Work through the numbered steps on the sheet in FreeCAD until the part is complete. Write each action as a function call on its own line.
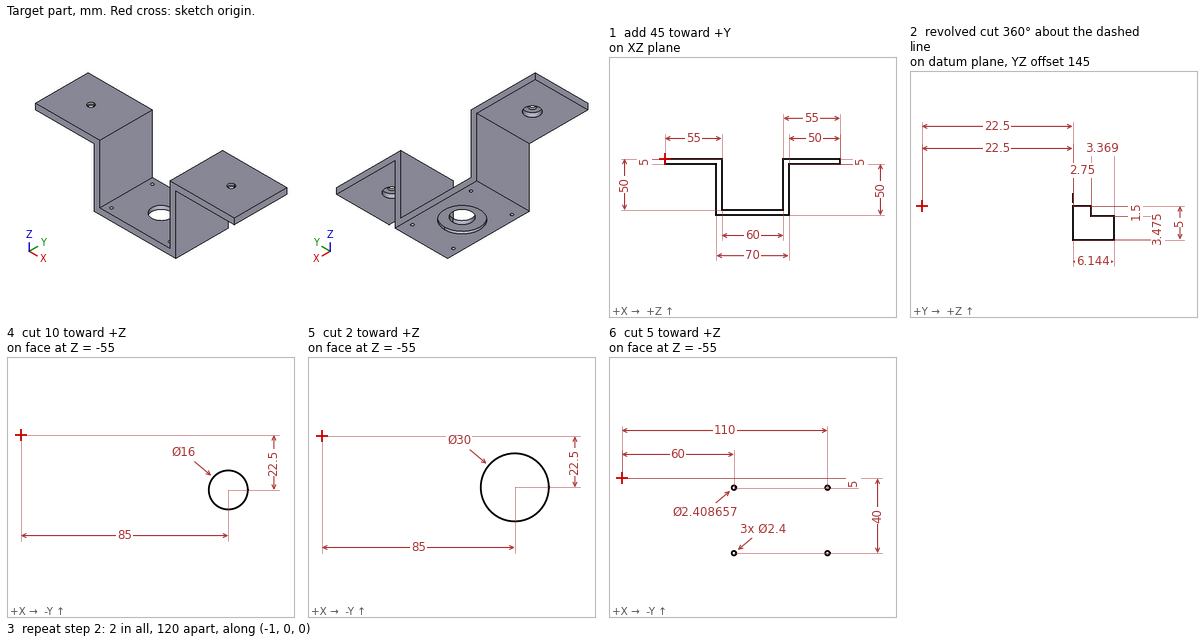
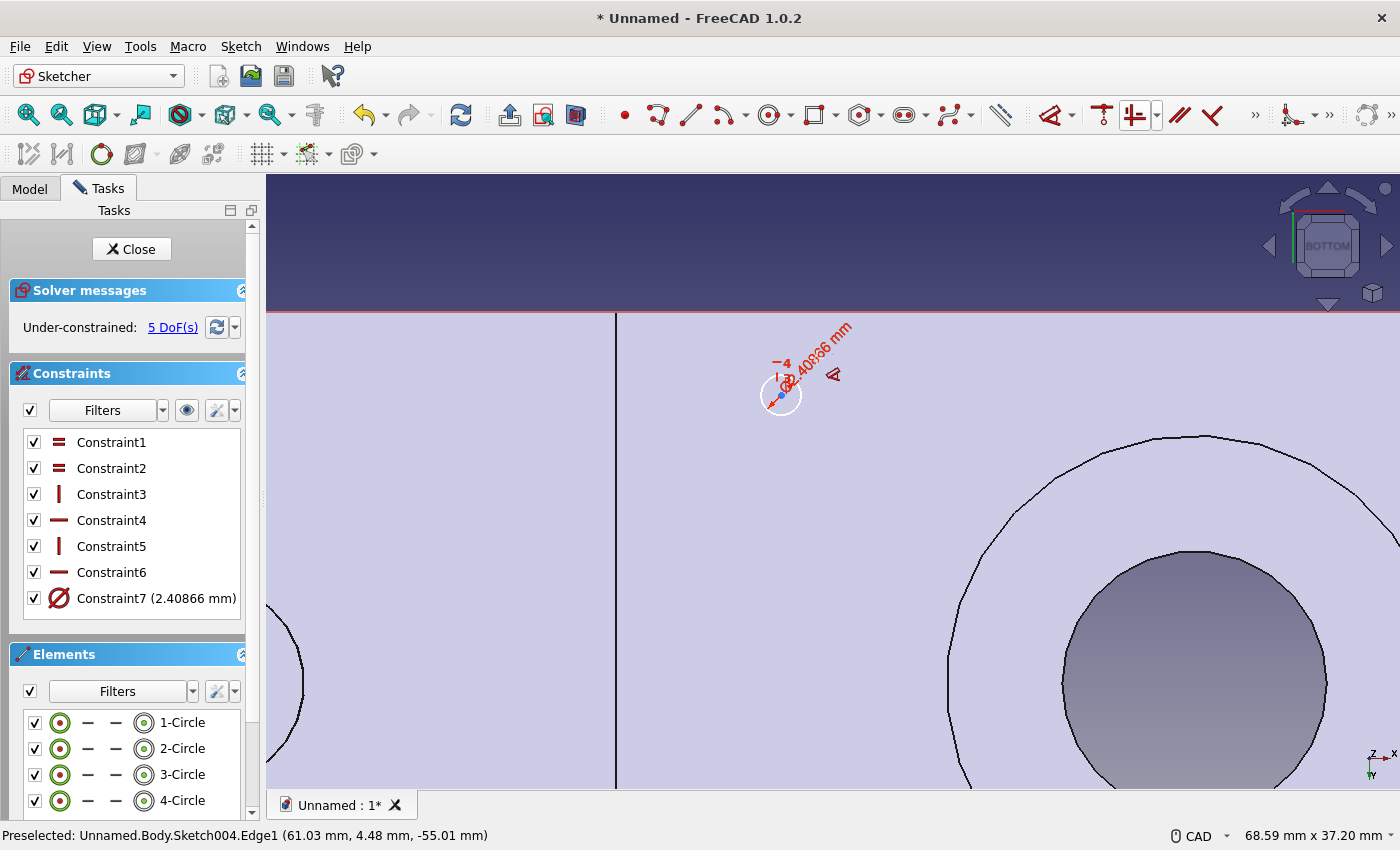
scroll(797, 382, down, 5)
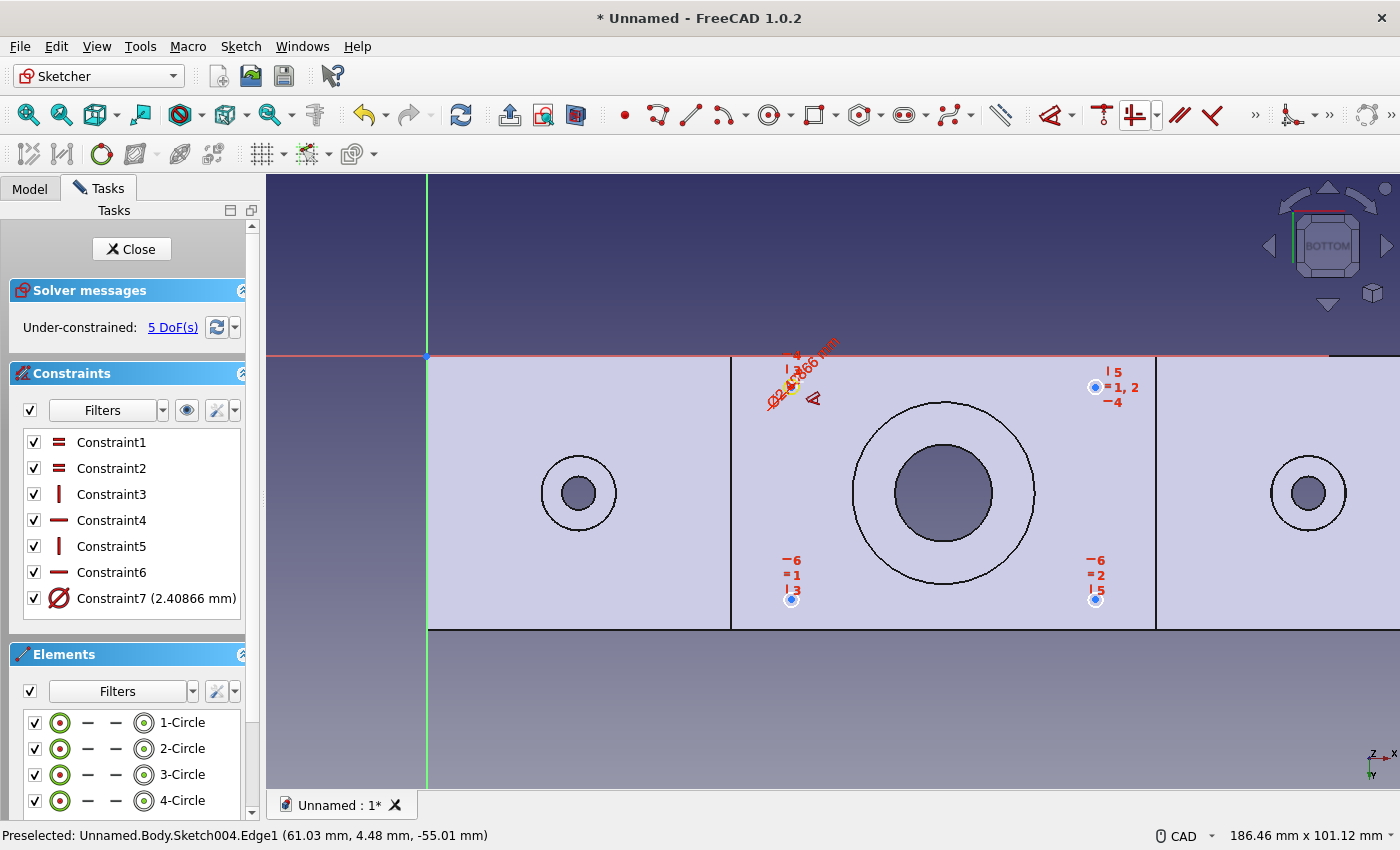
scroll(797, 595, up, 6)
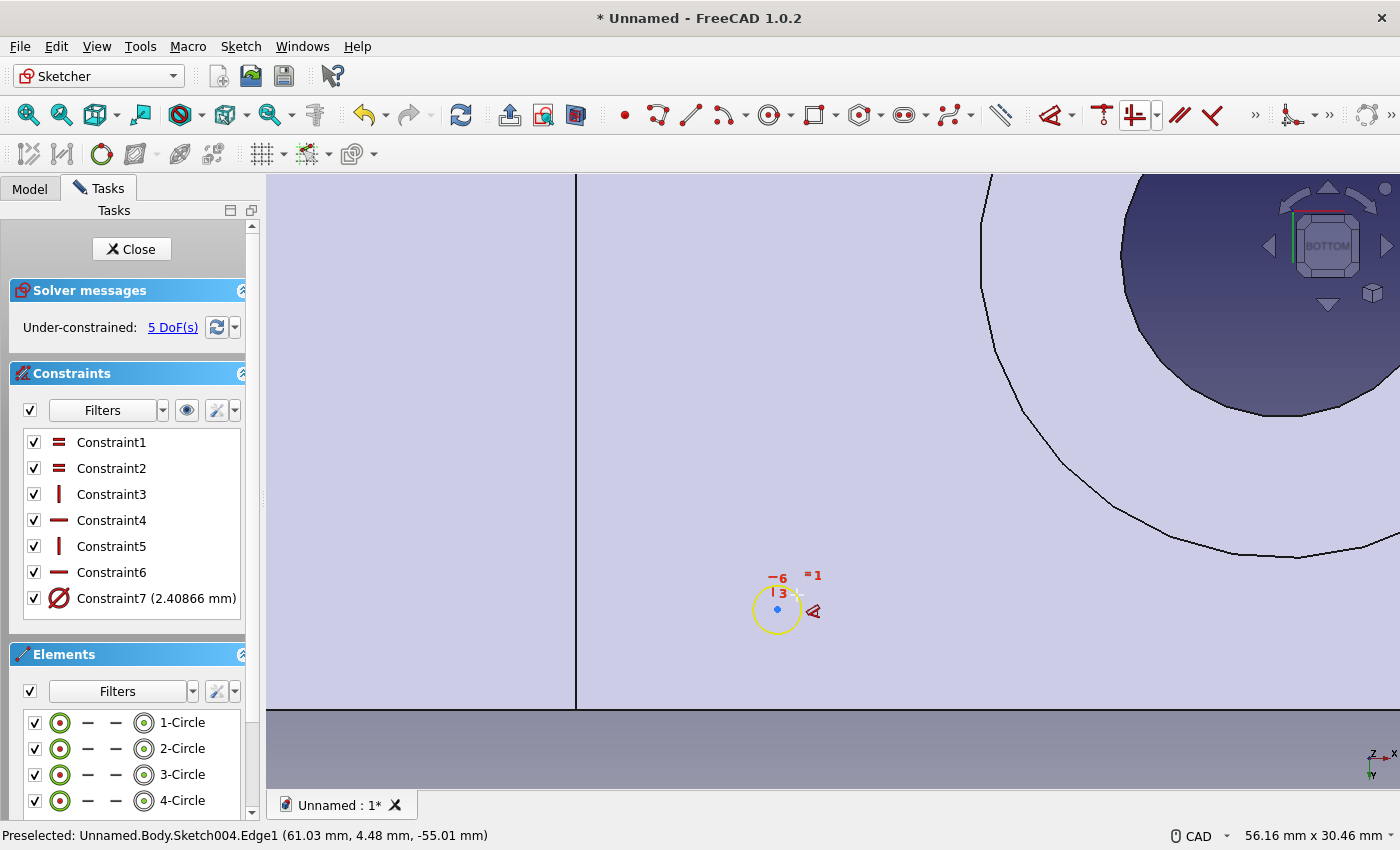
click(794, 593)
click(817, 570)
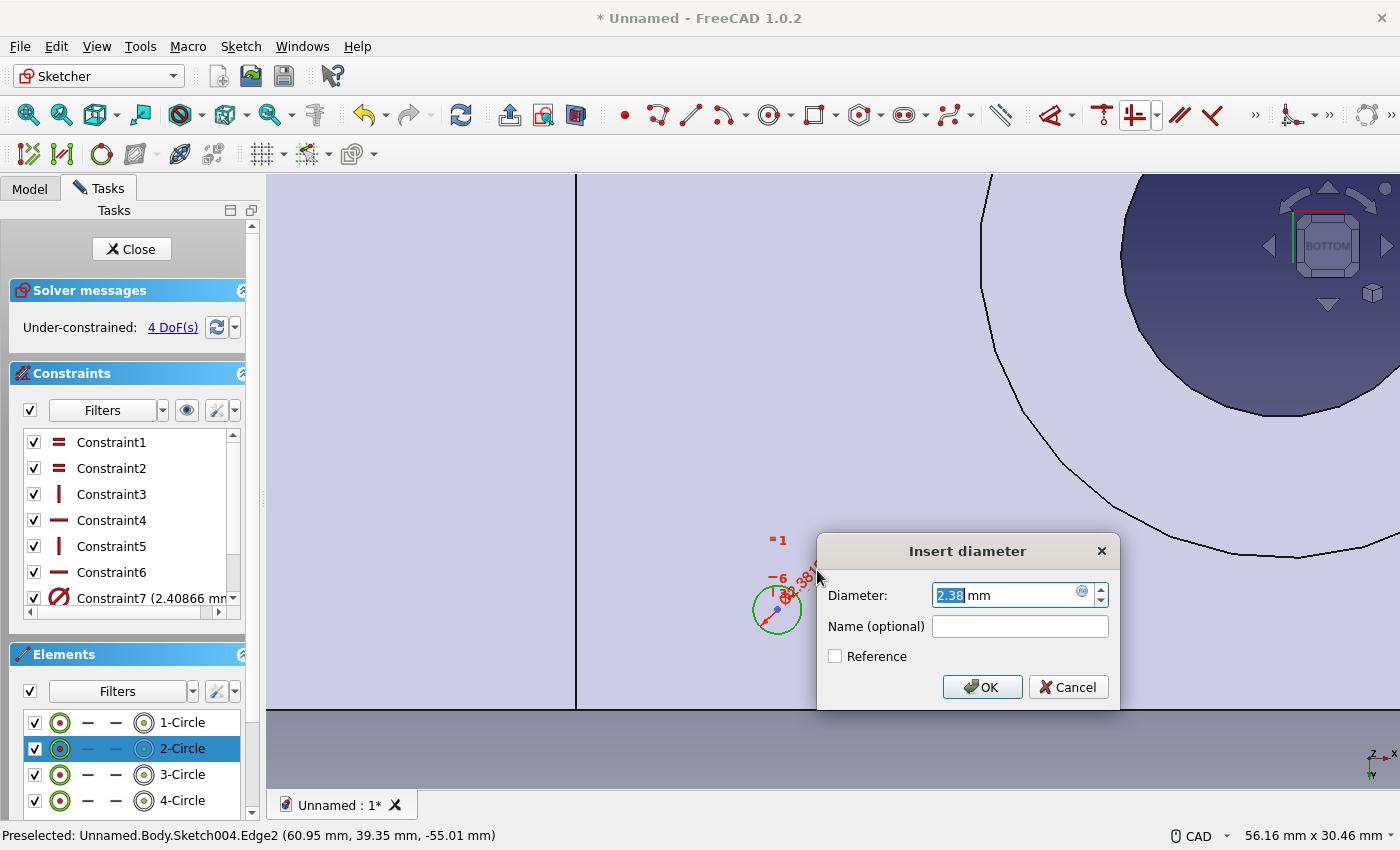
text(2.4)
key(Return)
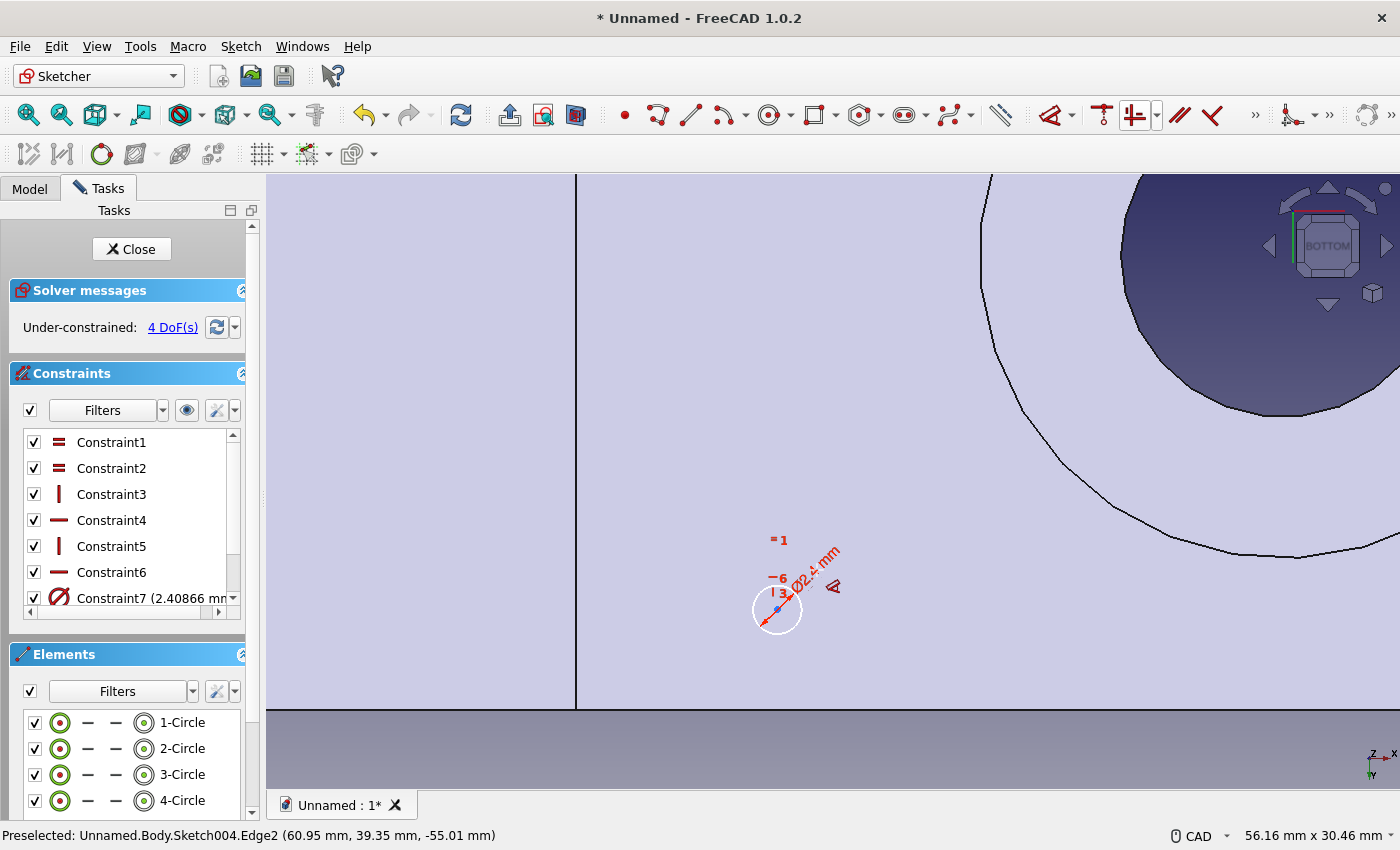
scroll(797, 596, down, 6)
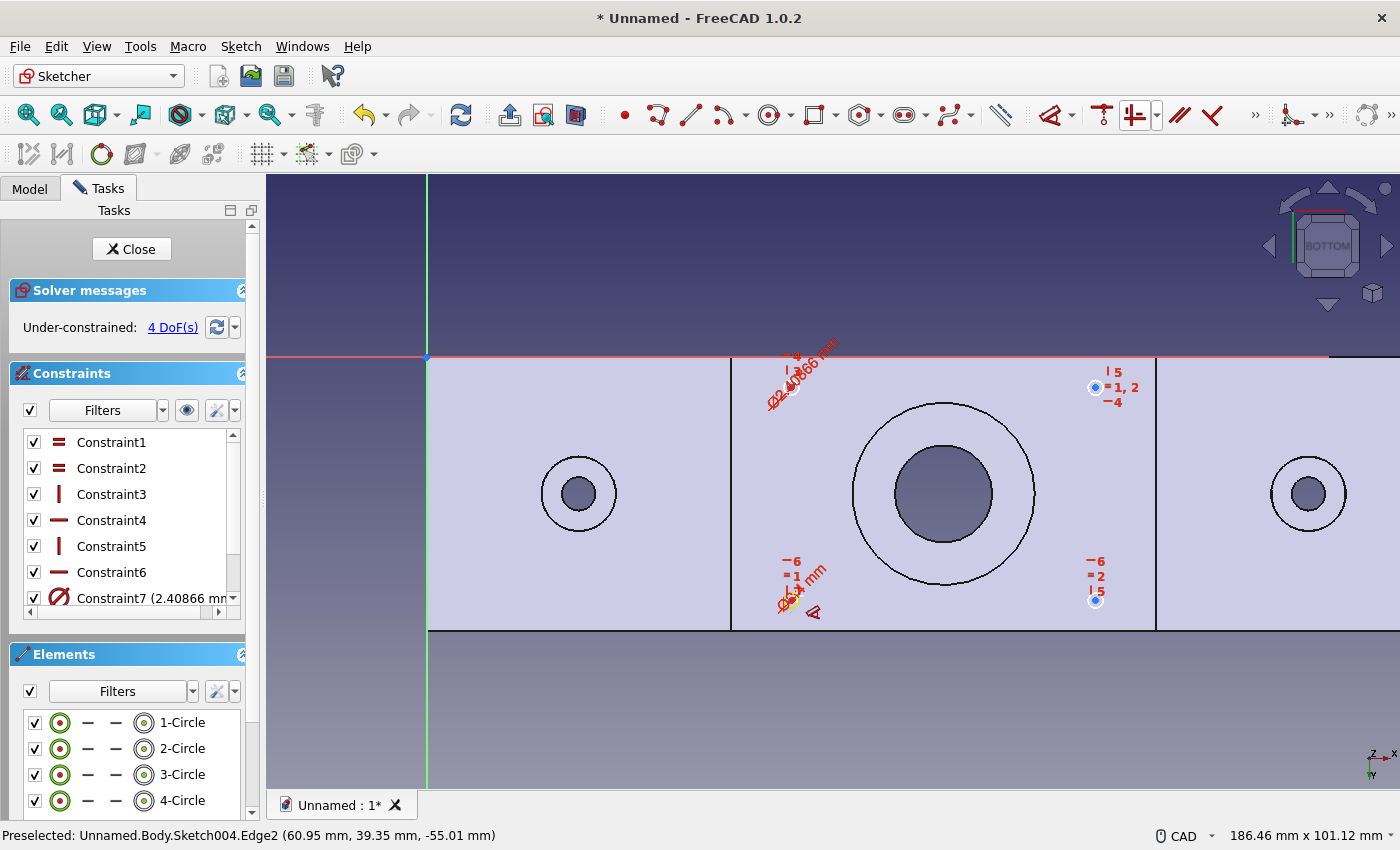
scroll(791, 388, up, 2)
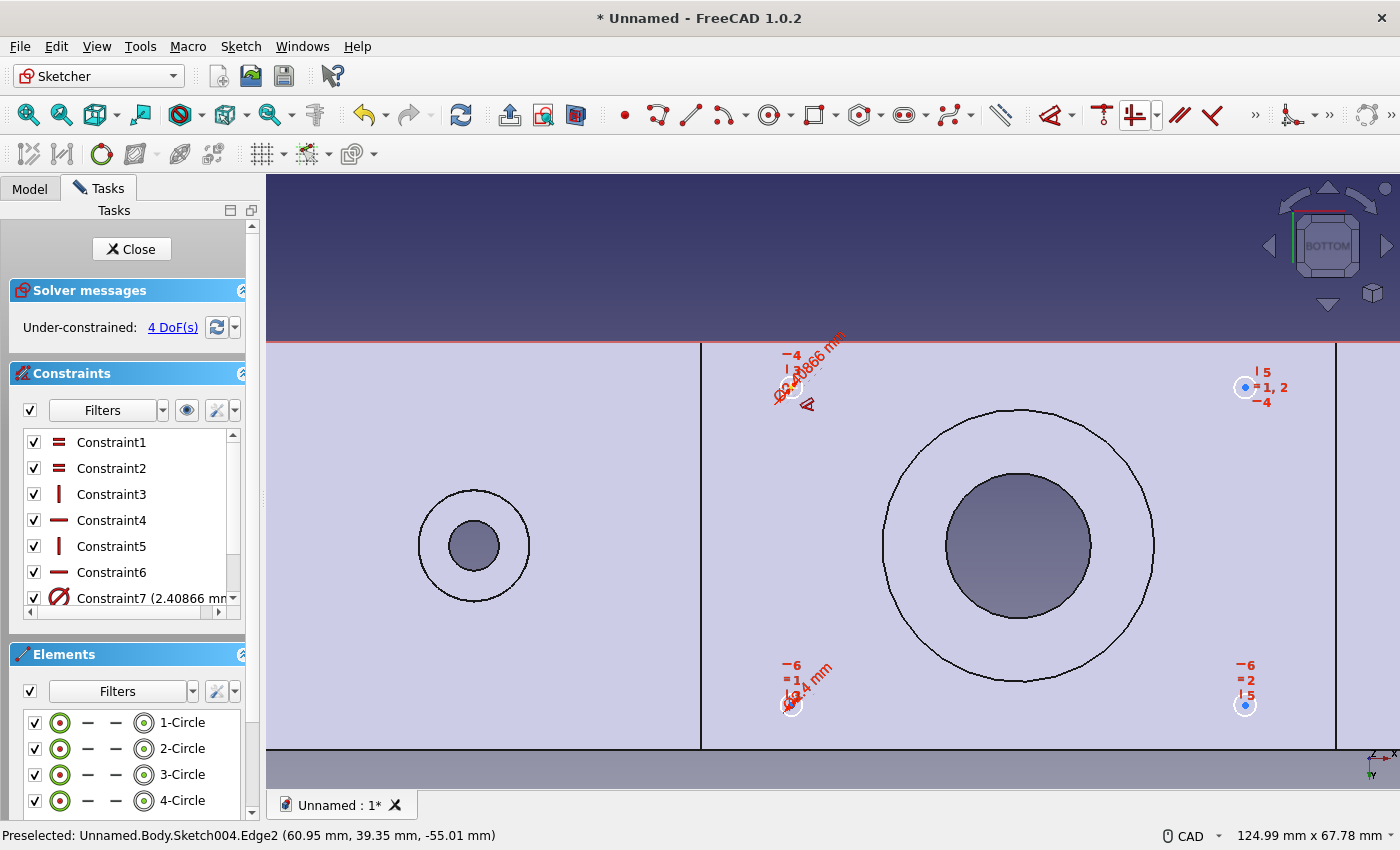
click(791, 388)
click(897, 365)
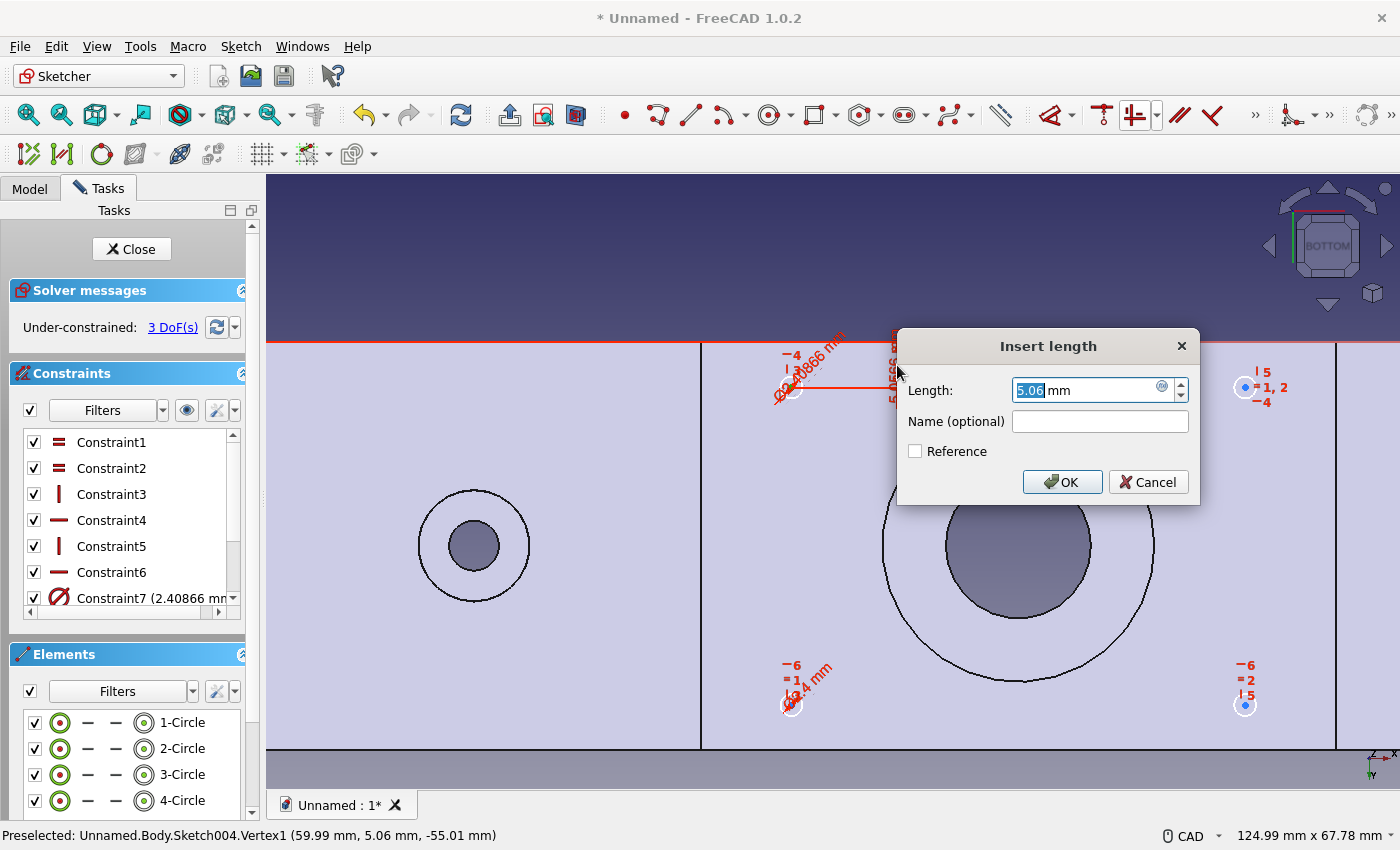
text(5)
key(Return)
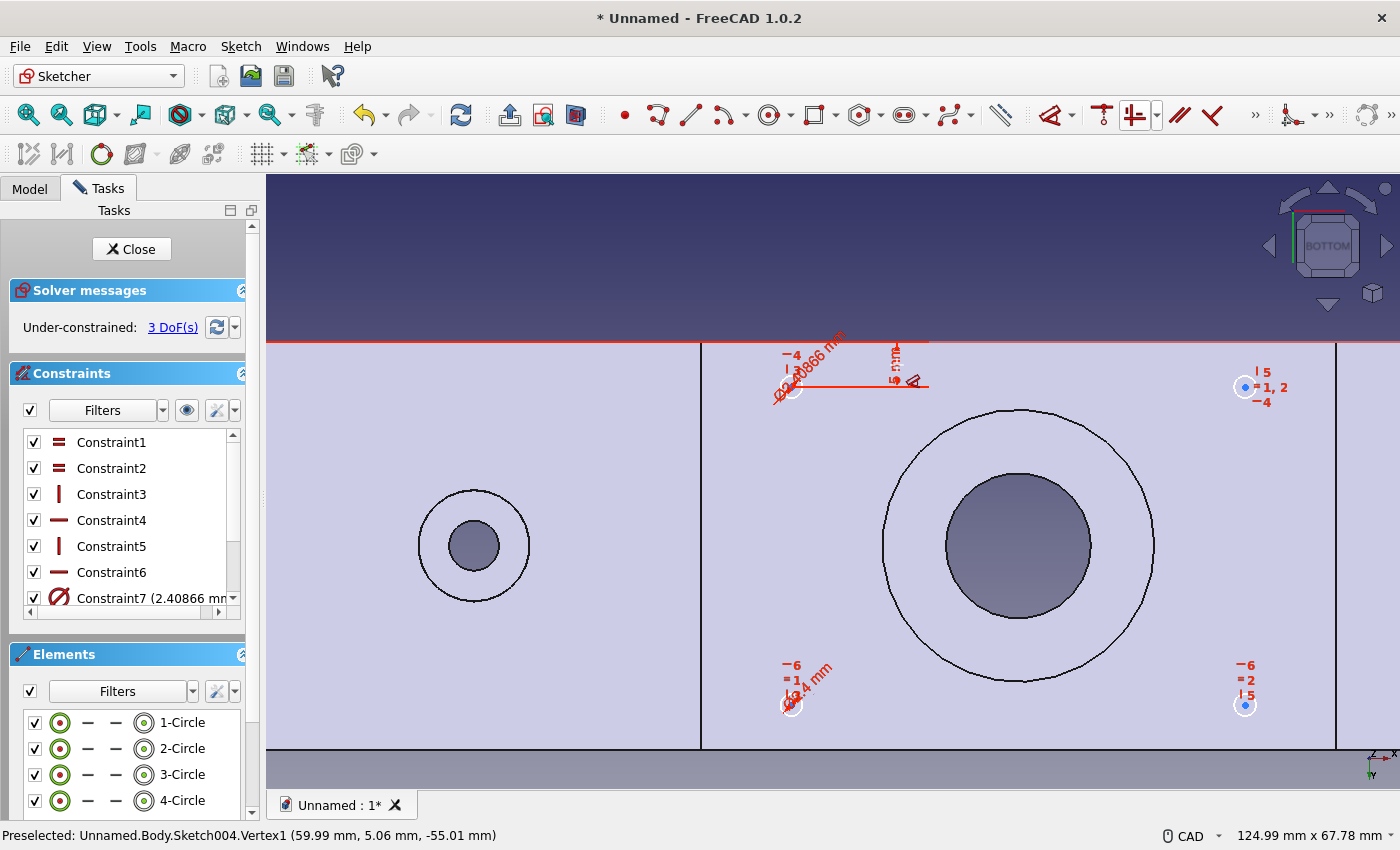
click(791, 387)
click(543, 308)